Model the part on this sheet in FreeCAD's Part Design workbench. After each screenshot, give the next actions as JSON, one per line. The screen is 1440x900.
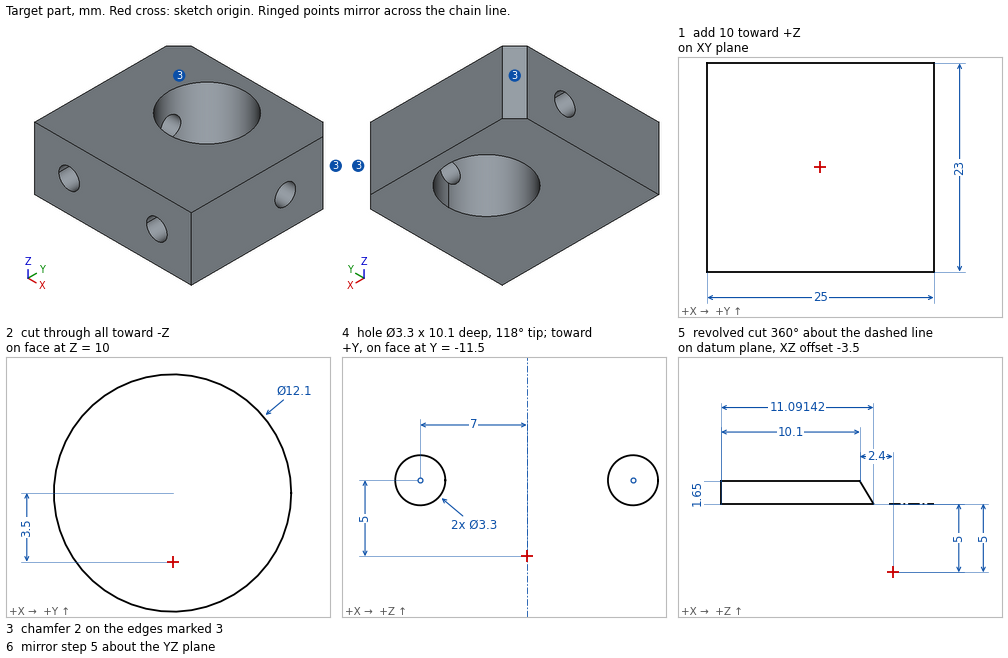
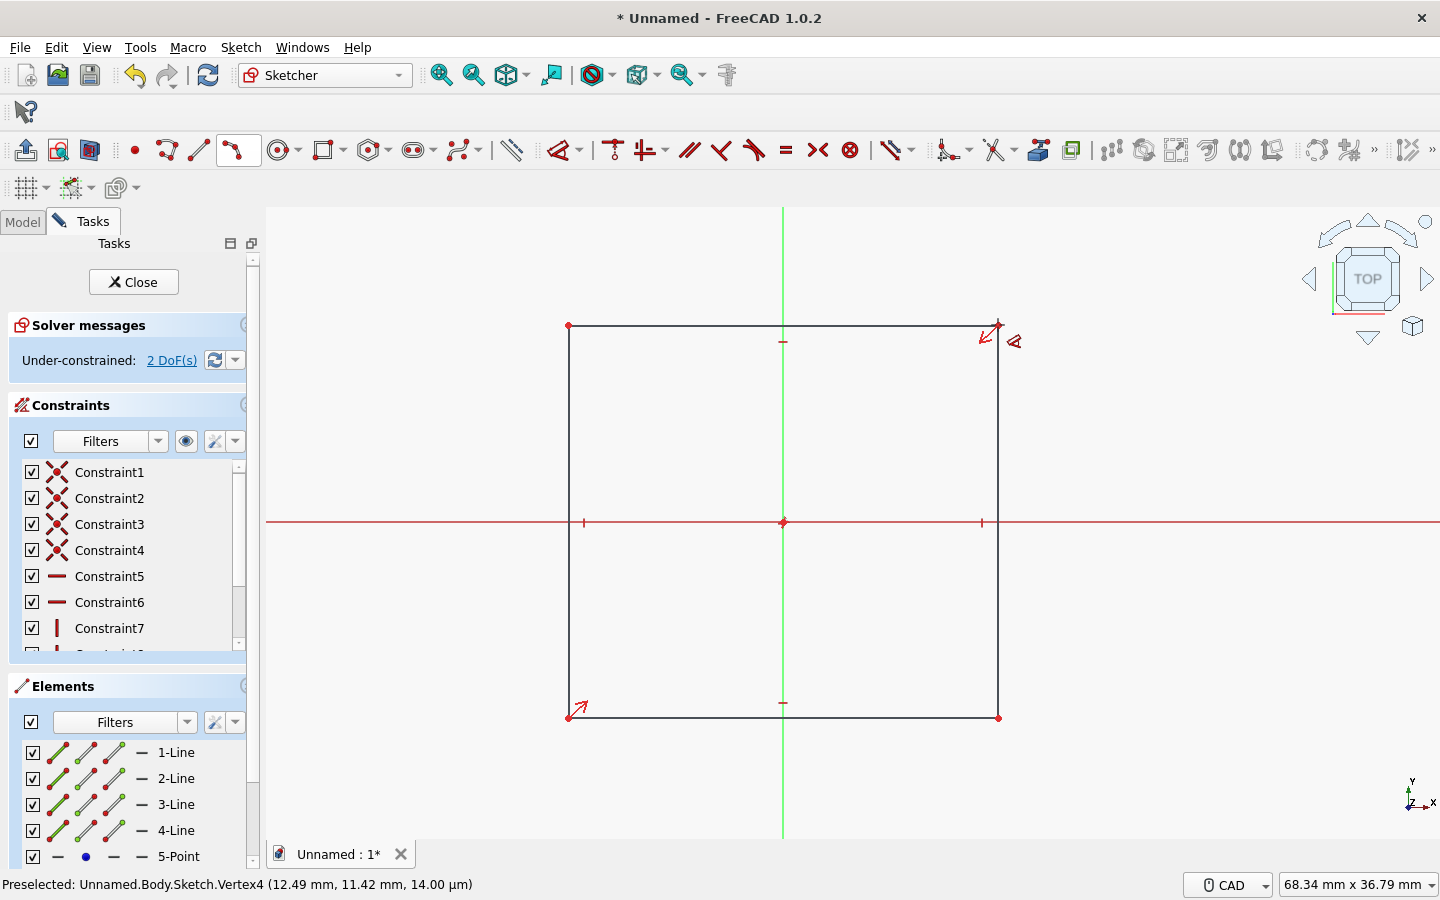
{"action": "left_click", "coordinate": [697, 718]}
{"action": "left_click", "coordinate": [685, 752]}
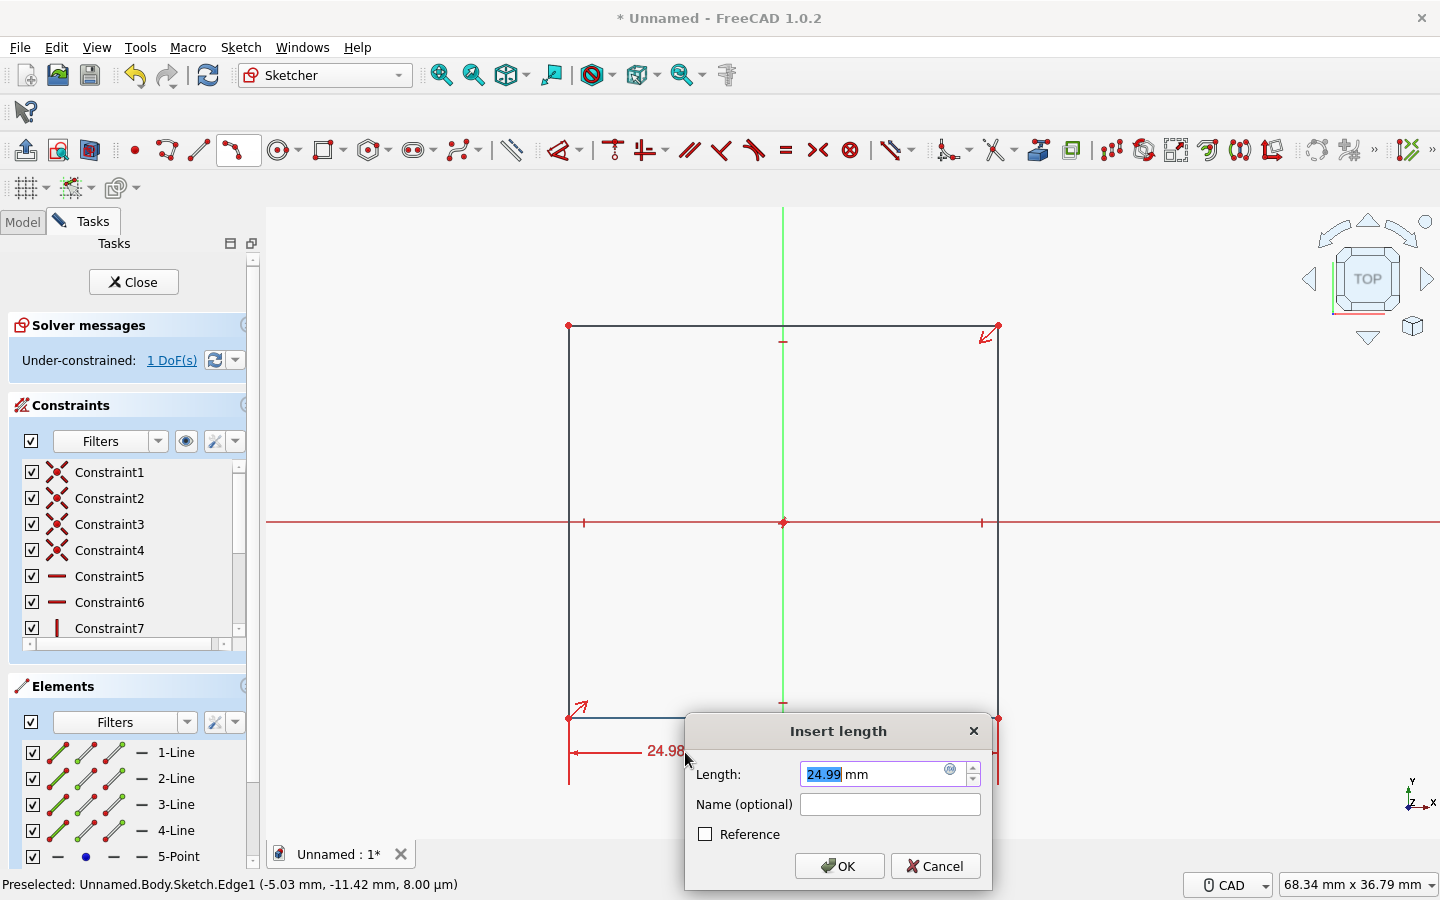
{"action": "type", "text": "25"}
{"action": "key", "text": "Return"}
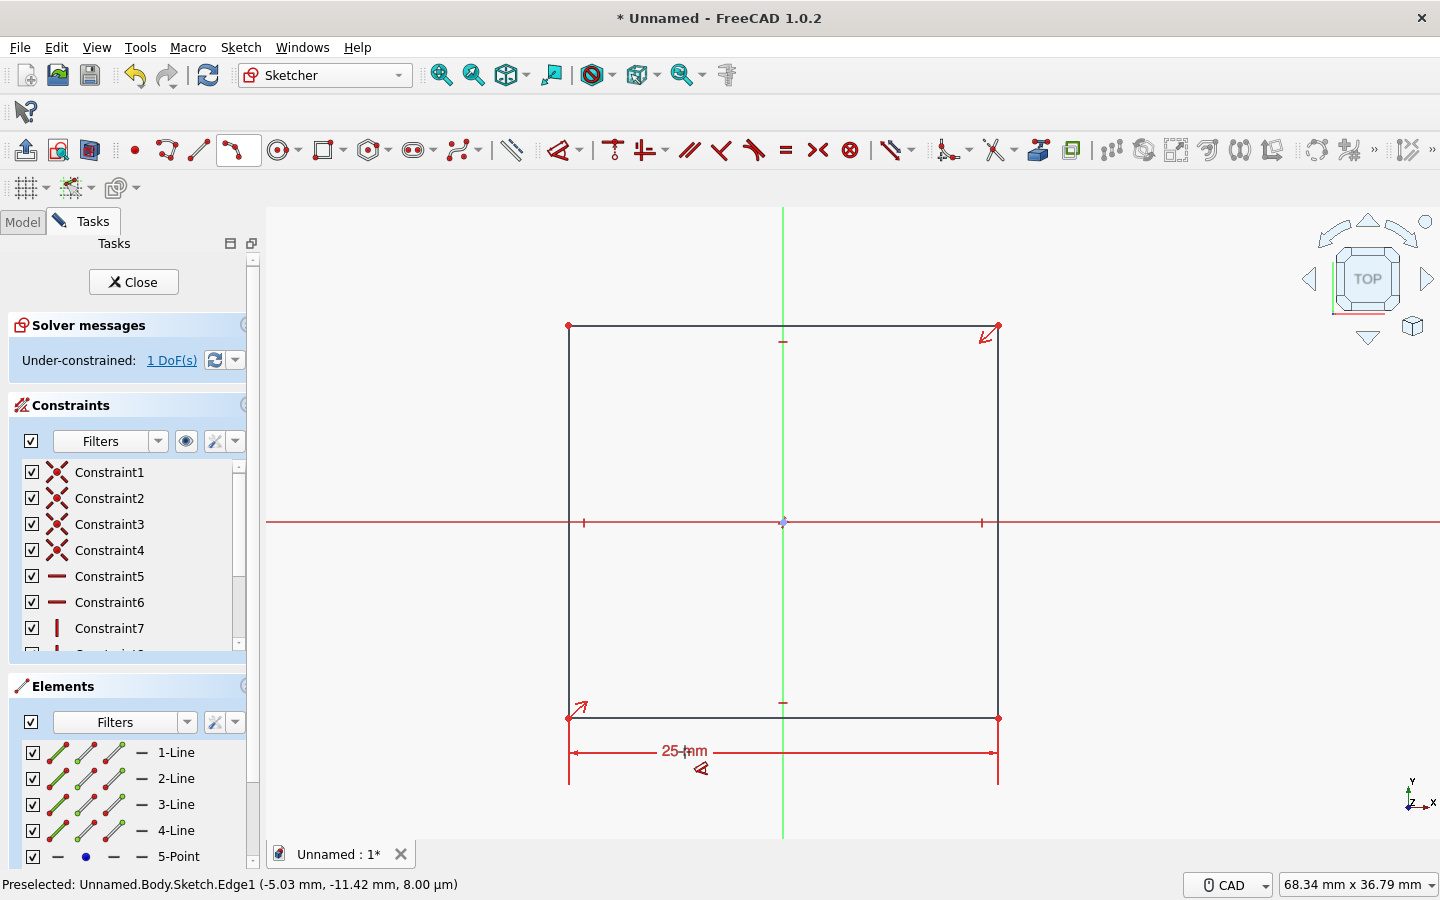
{"action": "left_click", "coordinate": [998, 601]}
{"action": "left_click", "coordinate": [1032, 432]}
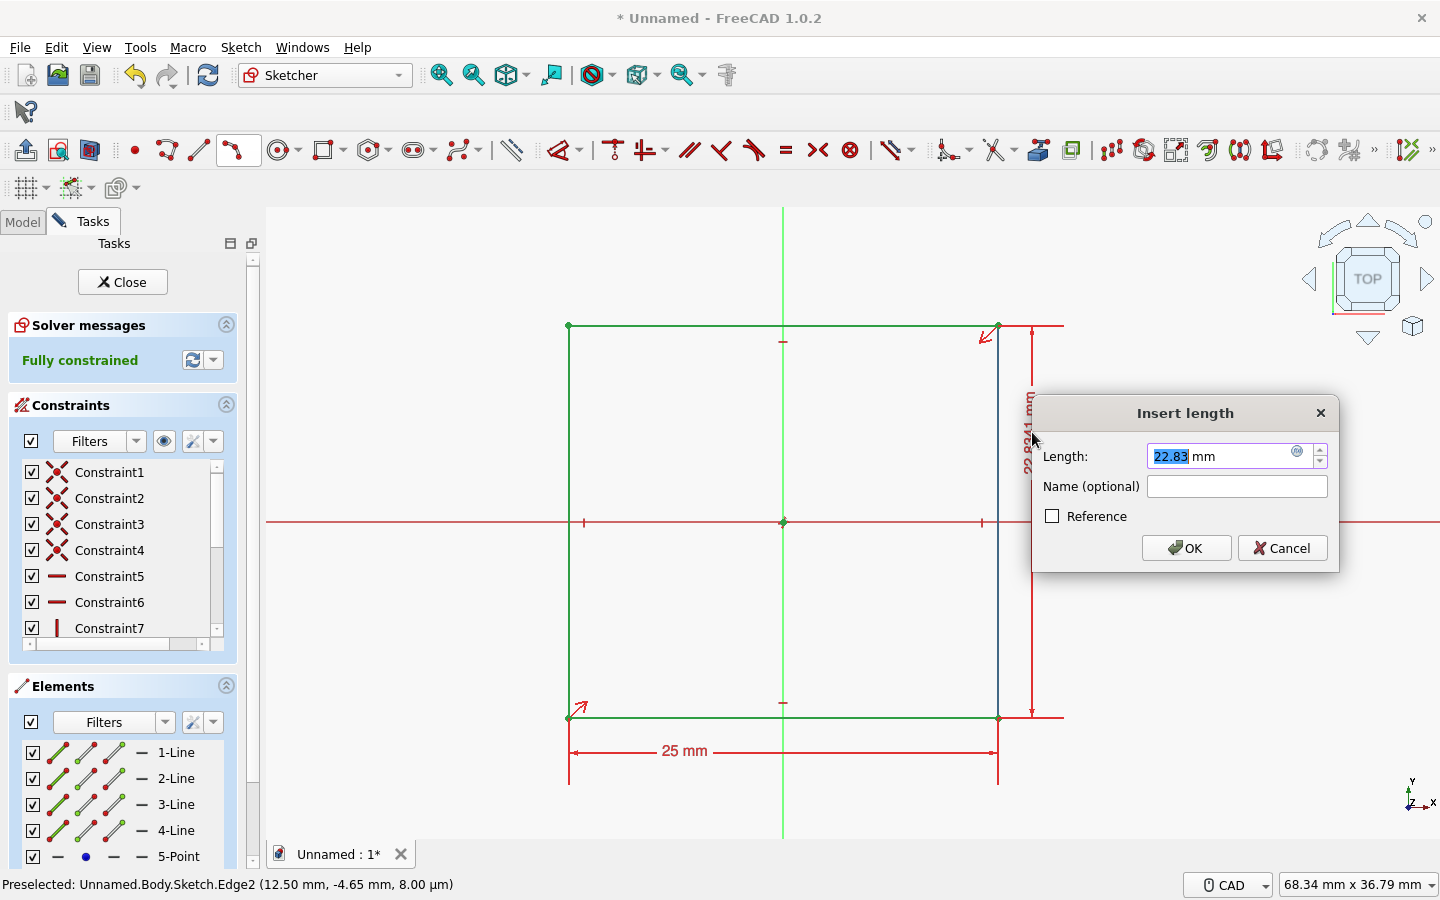
{"action": "type", "text": "23"}
{"action": "key", "text": "Return"}
{"action": "key", "text": "Escape"}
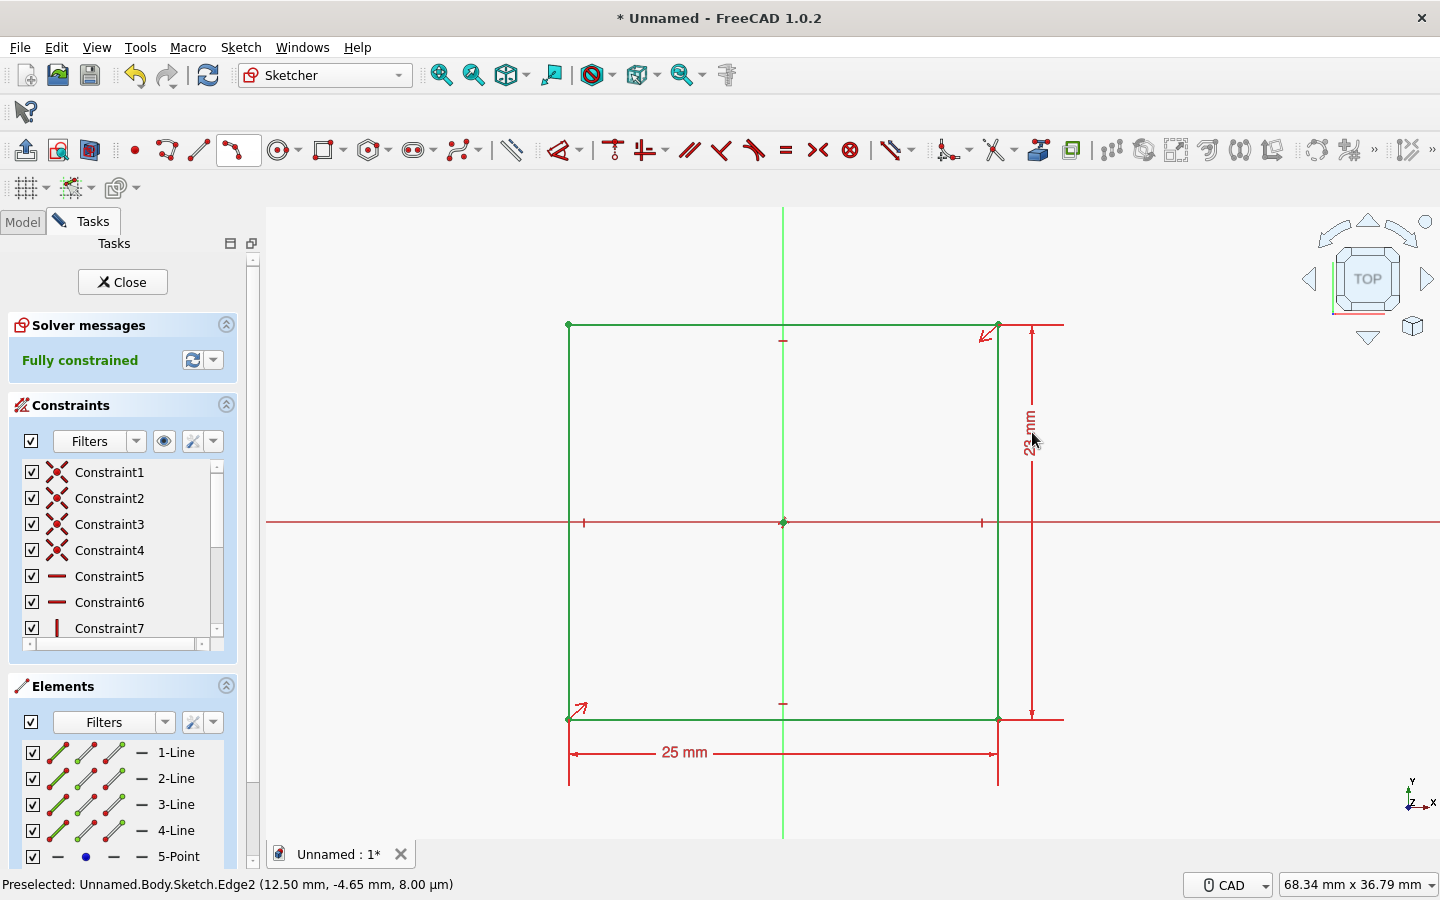
{"action": "left_click", "coordinate": [123, 282]}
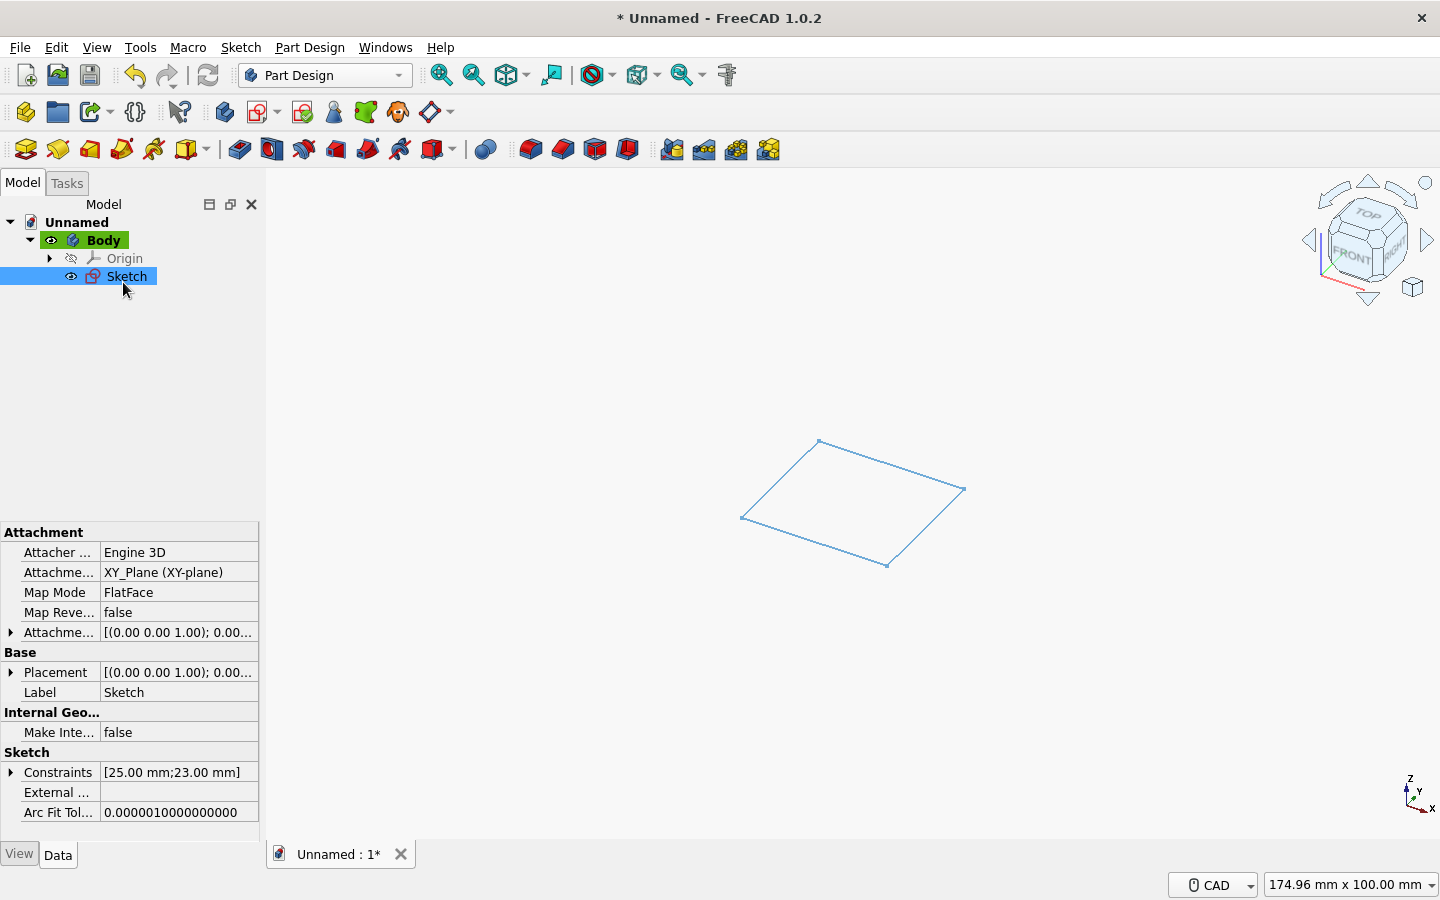
{"action": "left_click", "coordinate": [26, 150]}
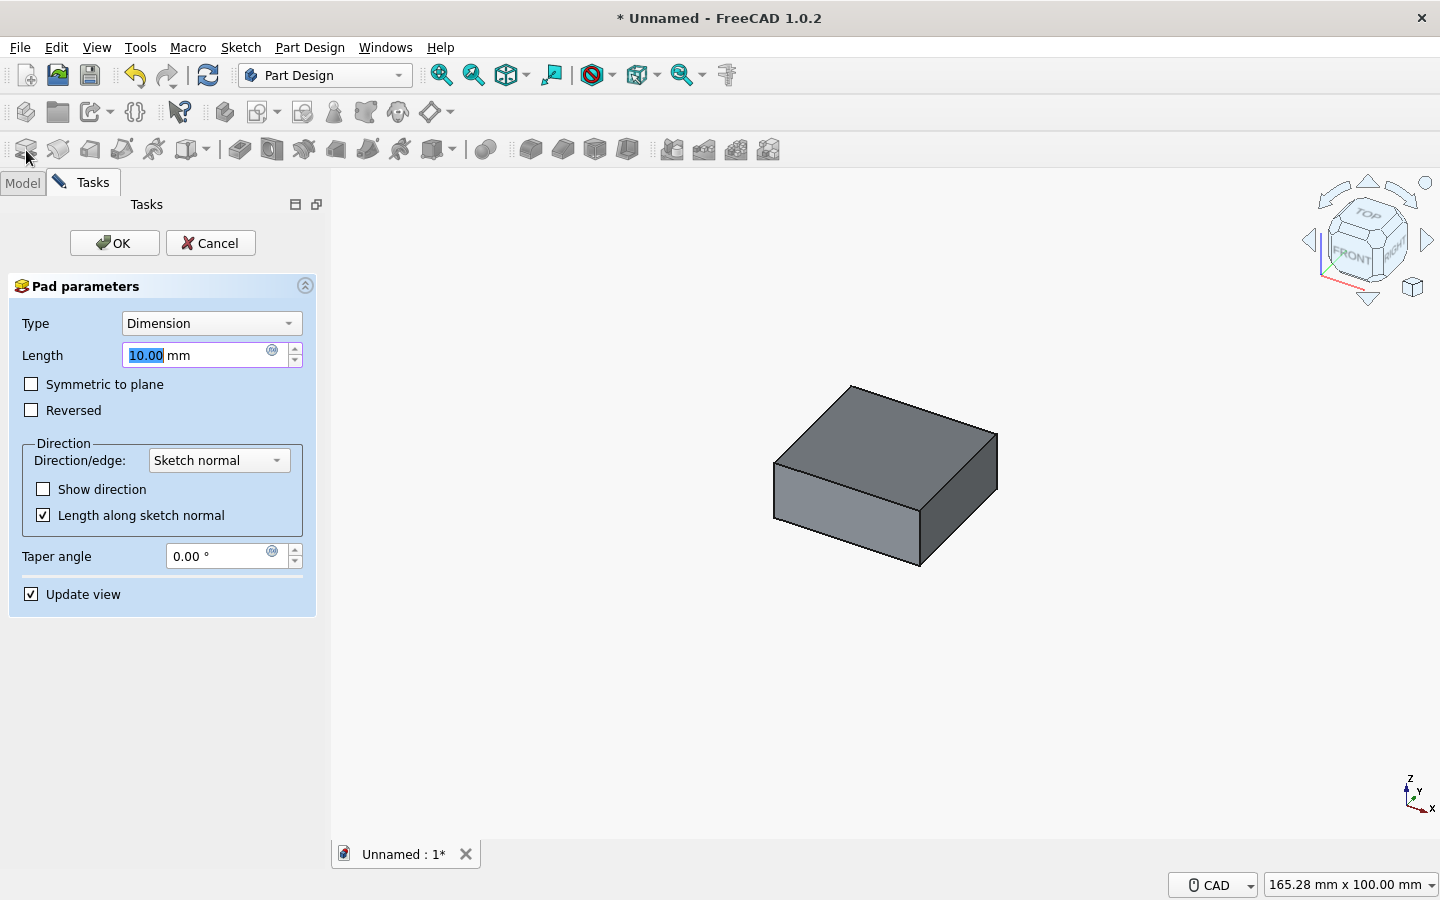
{"action": "type", "text": "10"}
{"action": "key", "text": "Tab"}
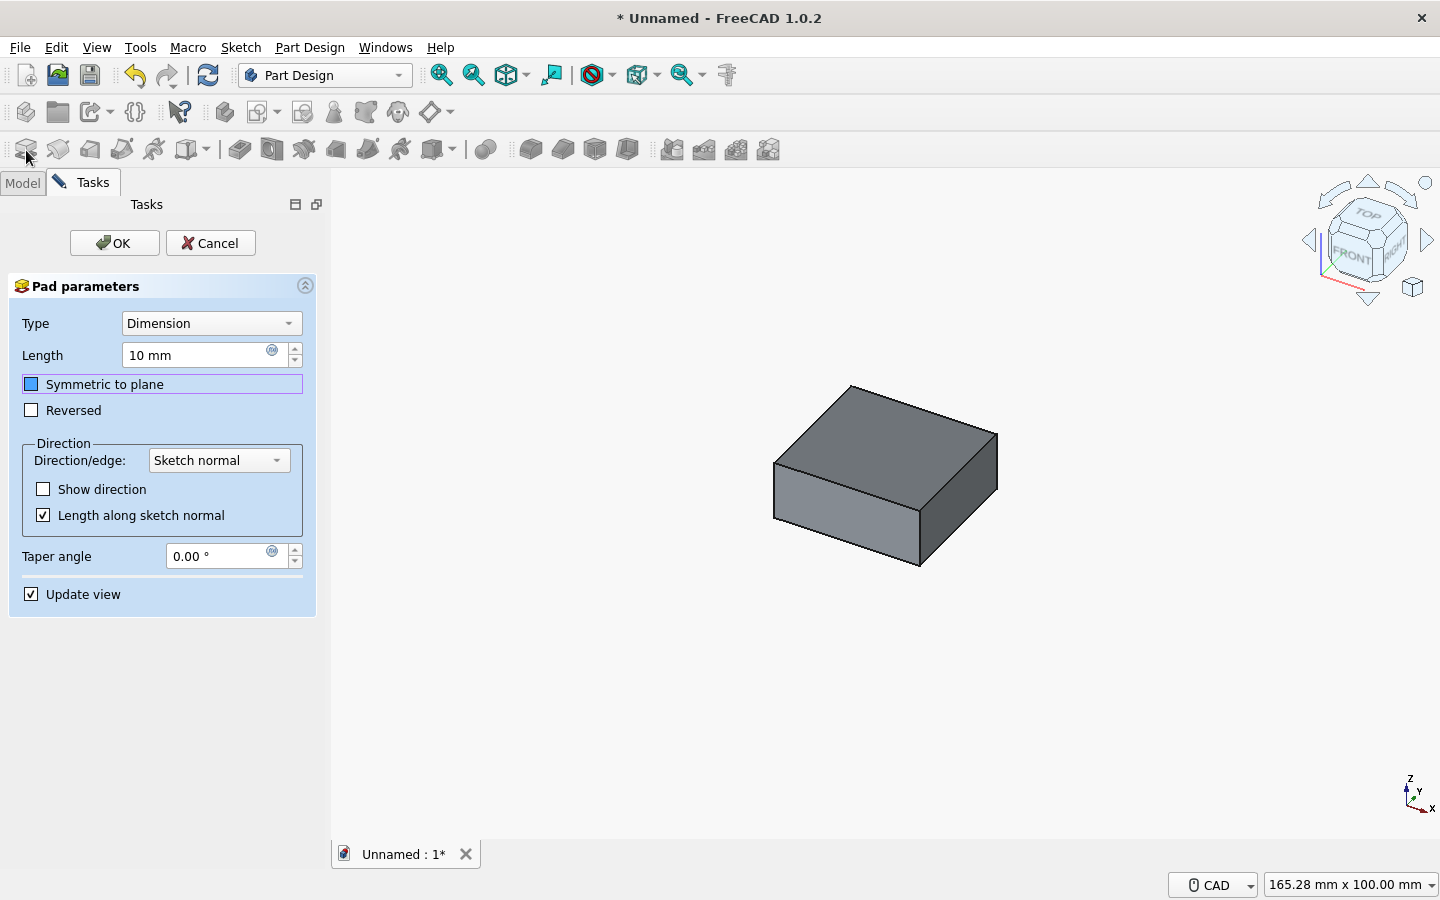
{"action": "left_click", "coordinate": [115, 243]}